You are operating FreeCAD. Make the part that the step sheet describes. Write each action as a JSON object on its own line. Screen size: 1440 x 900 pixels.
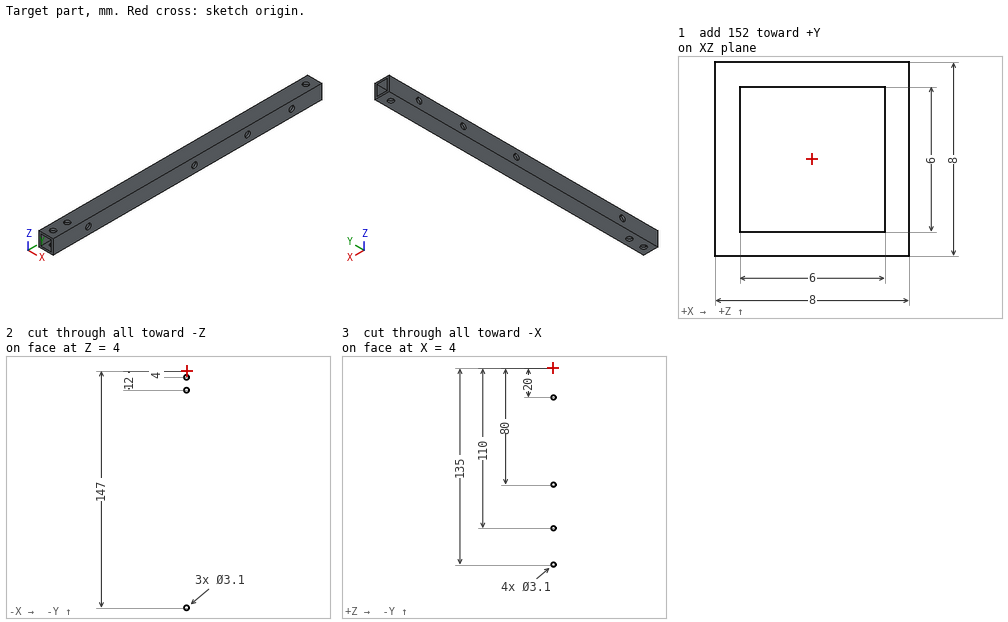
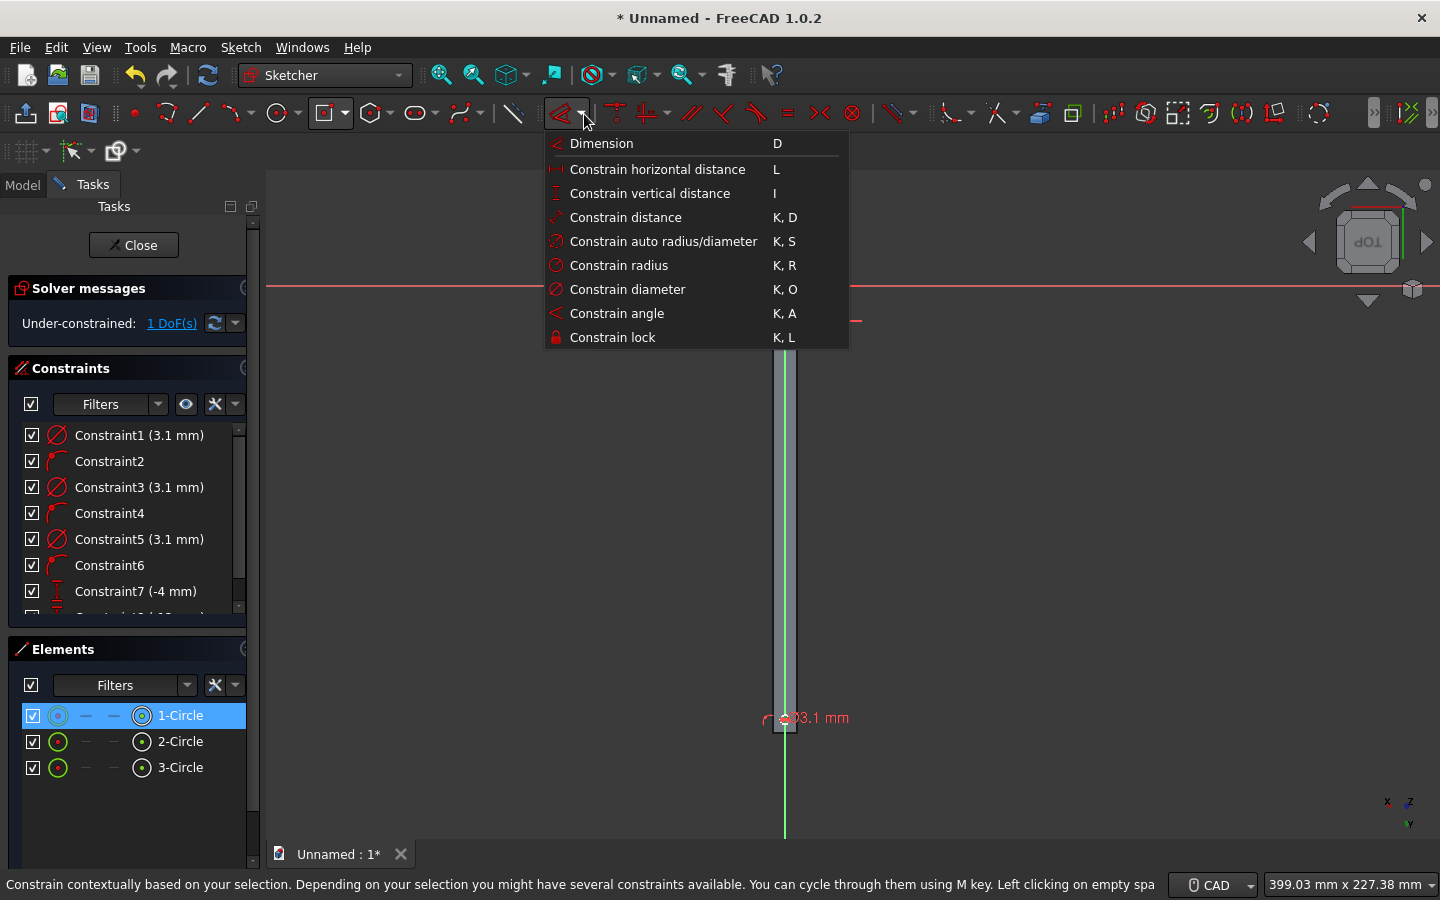
{"action": "left_click", "coordinate": [697, 193]}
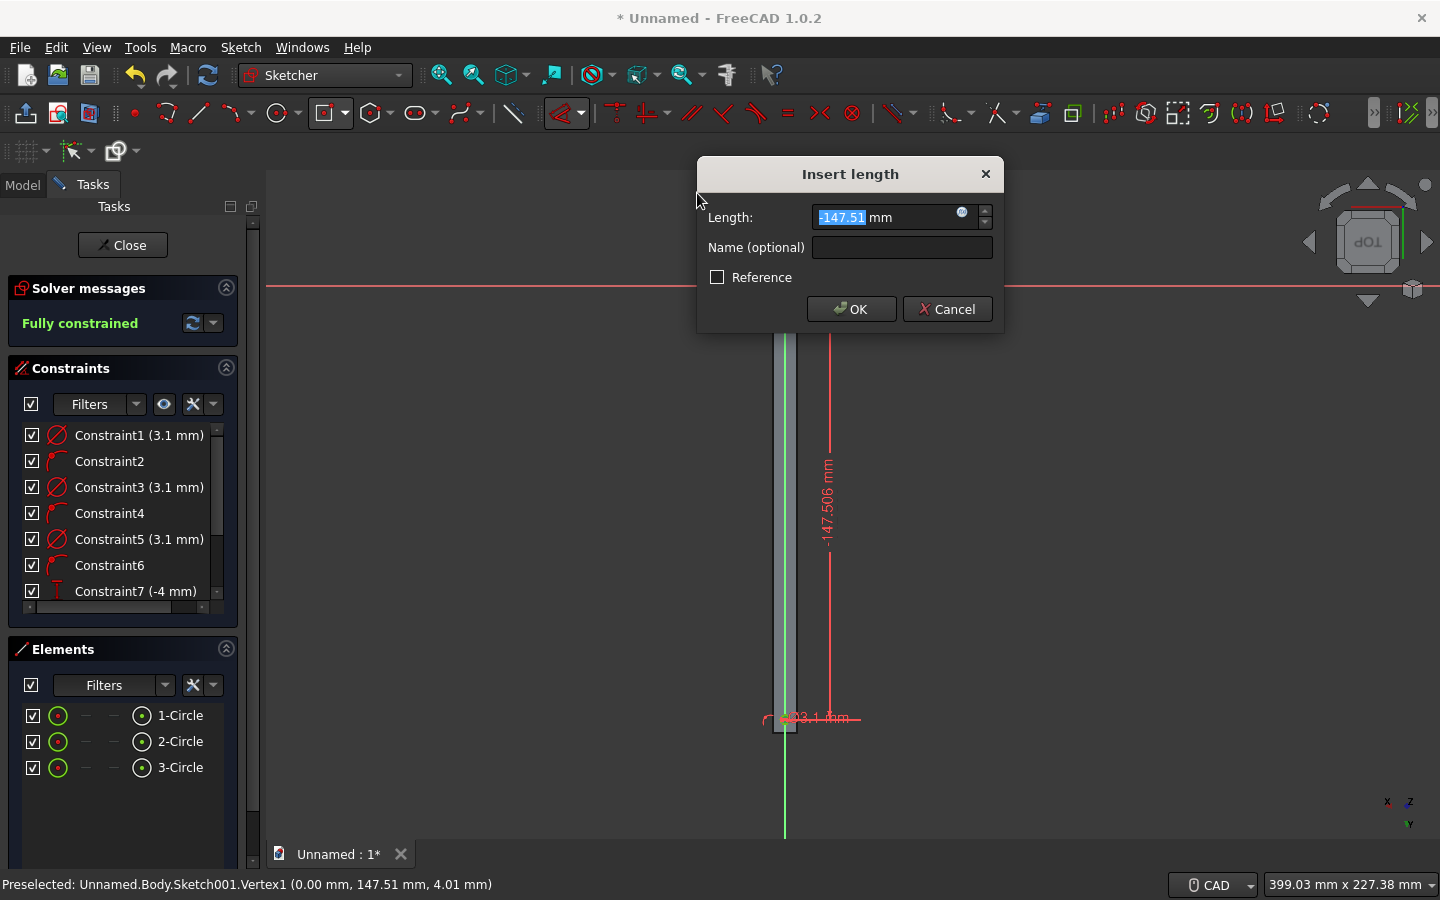
{"action": "type", "text": "-147"}
{"action": "key", "text": "Return"}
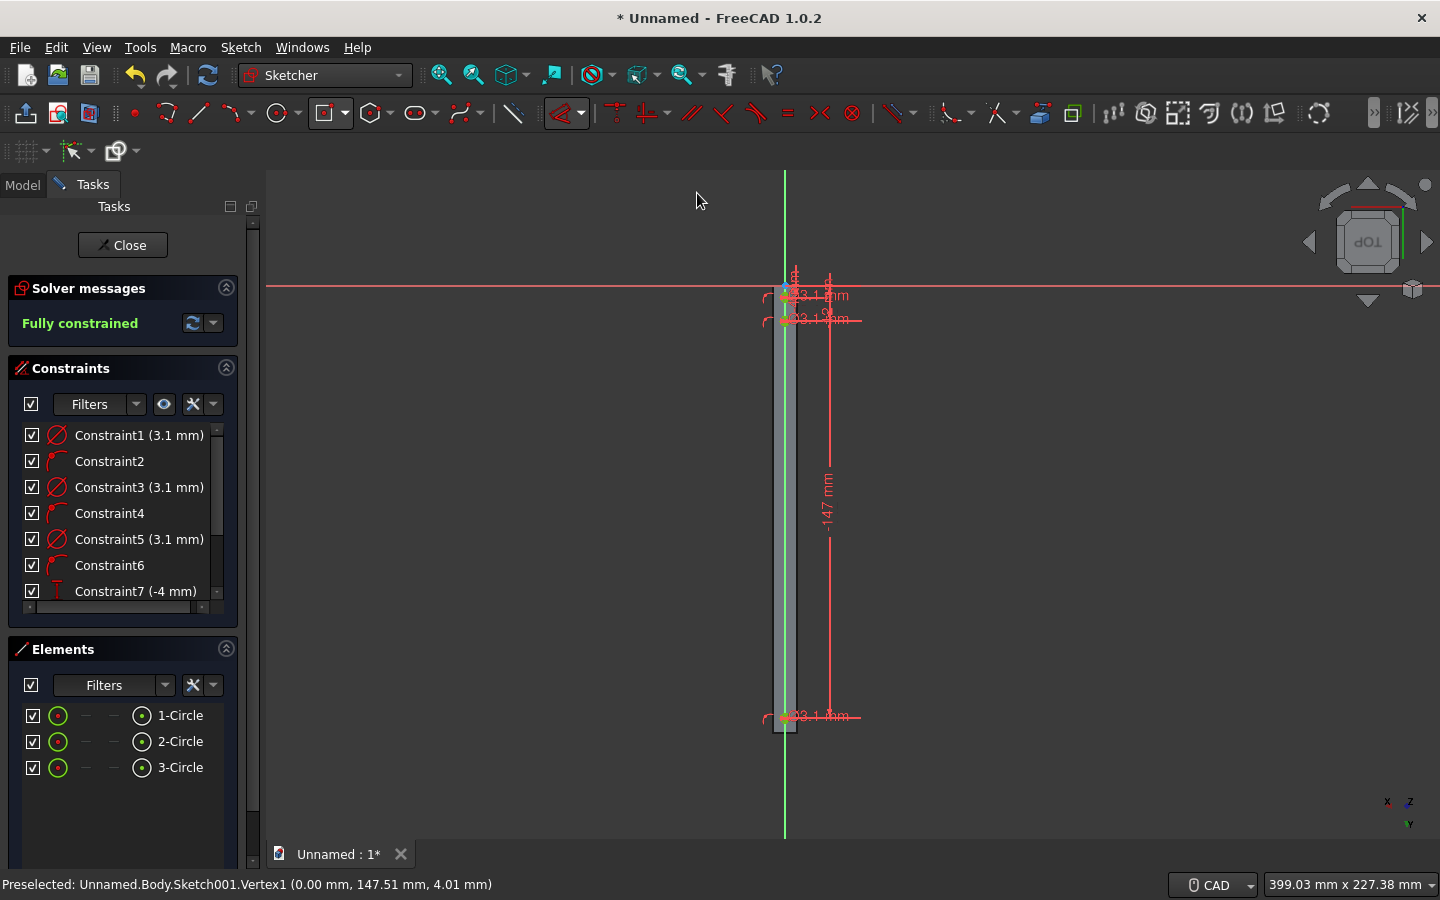
{"action": "left_click", "coordinate": [123, 245]}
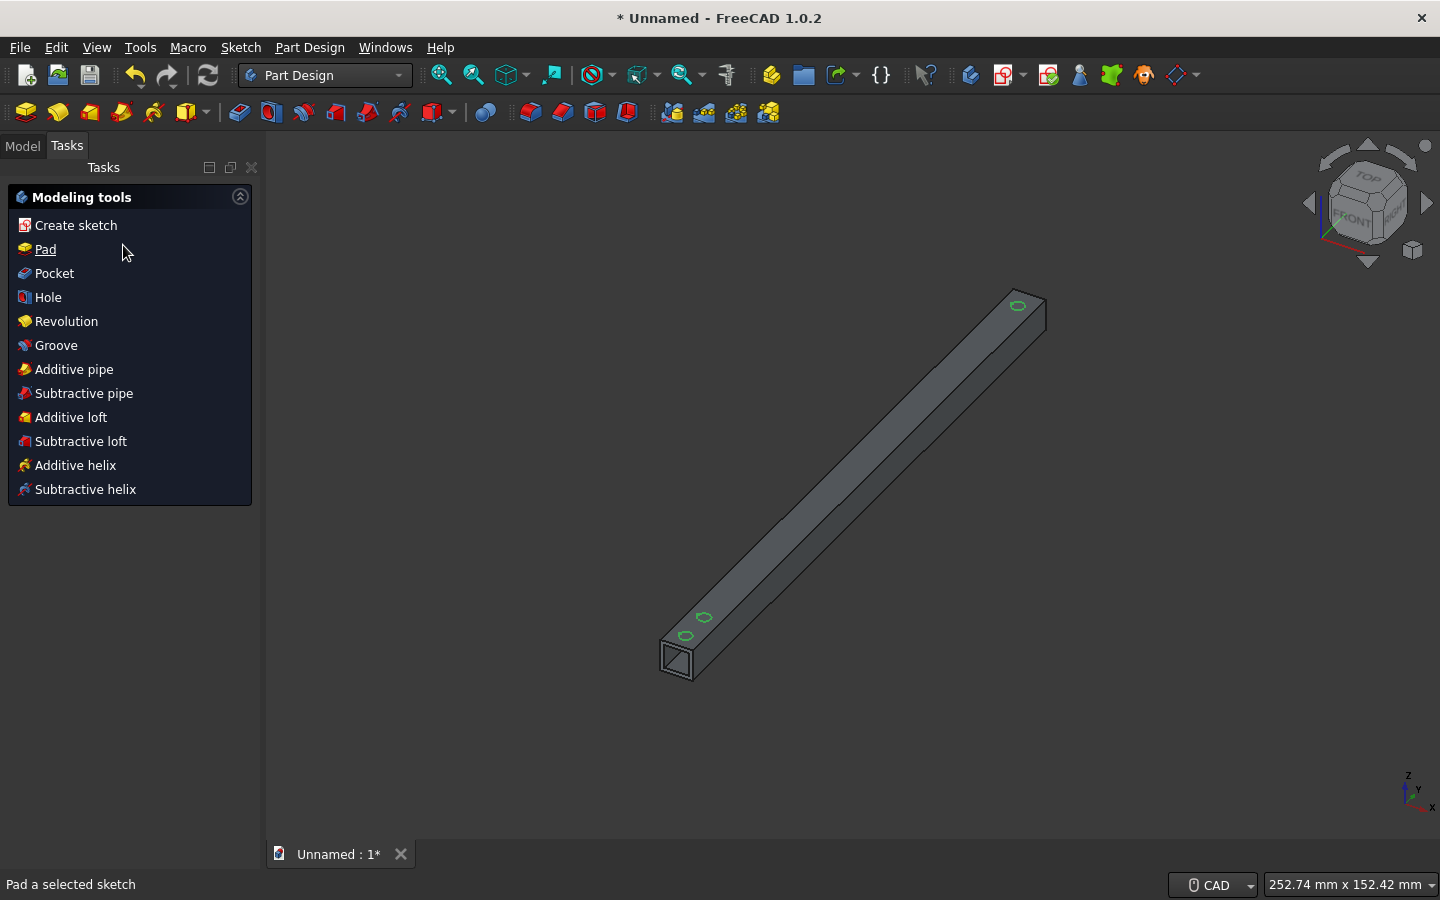
{"action": "left_click", "coordinate": [240, 112]}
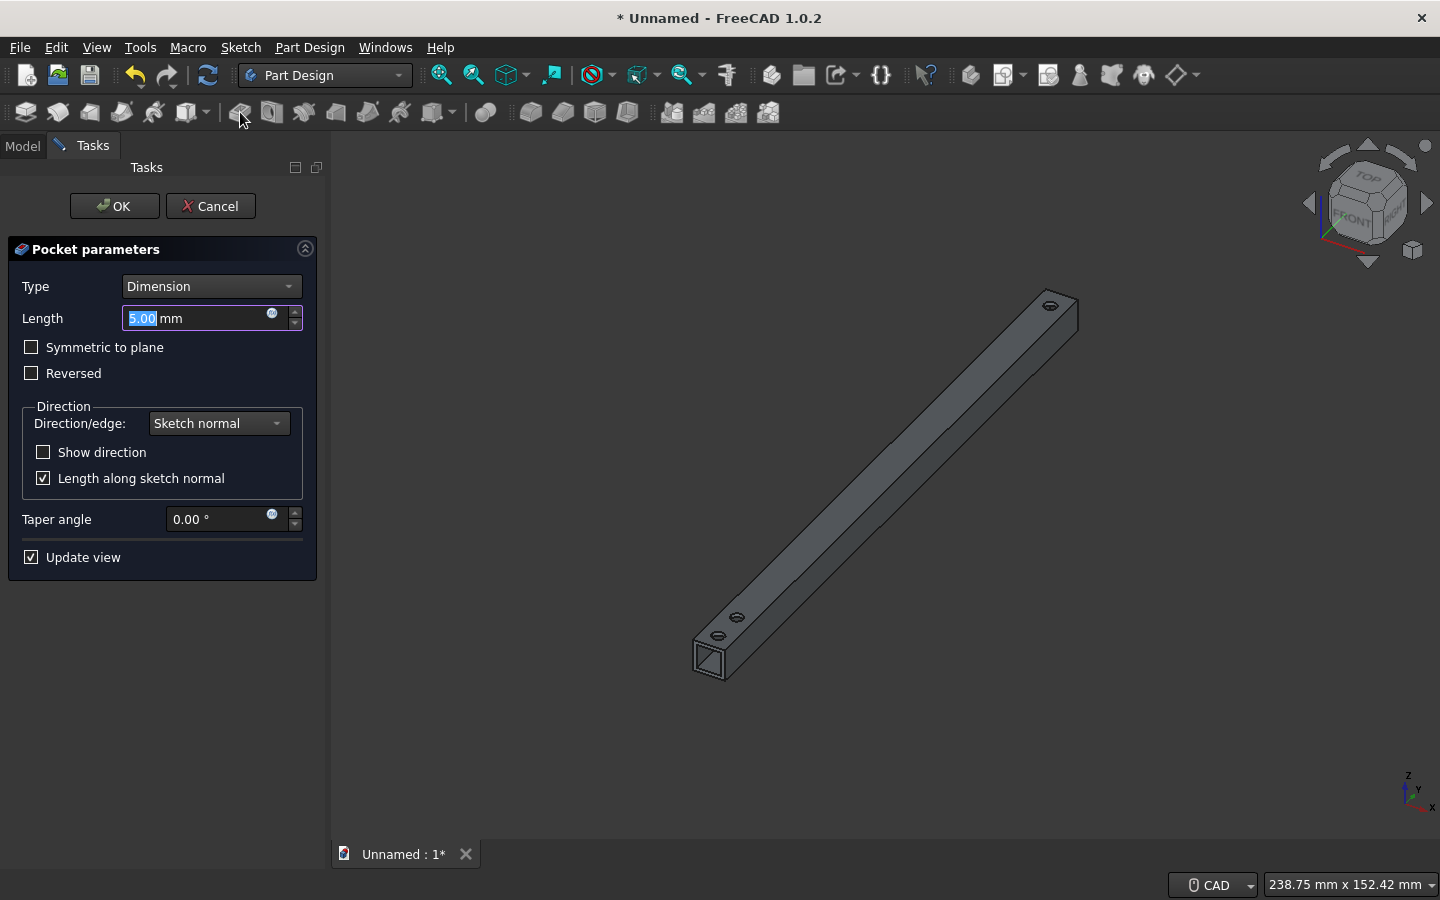
{"action": "left_click", "coordinate": [212, 286]}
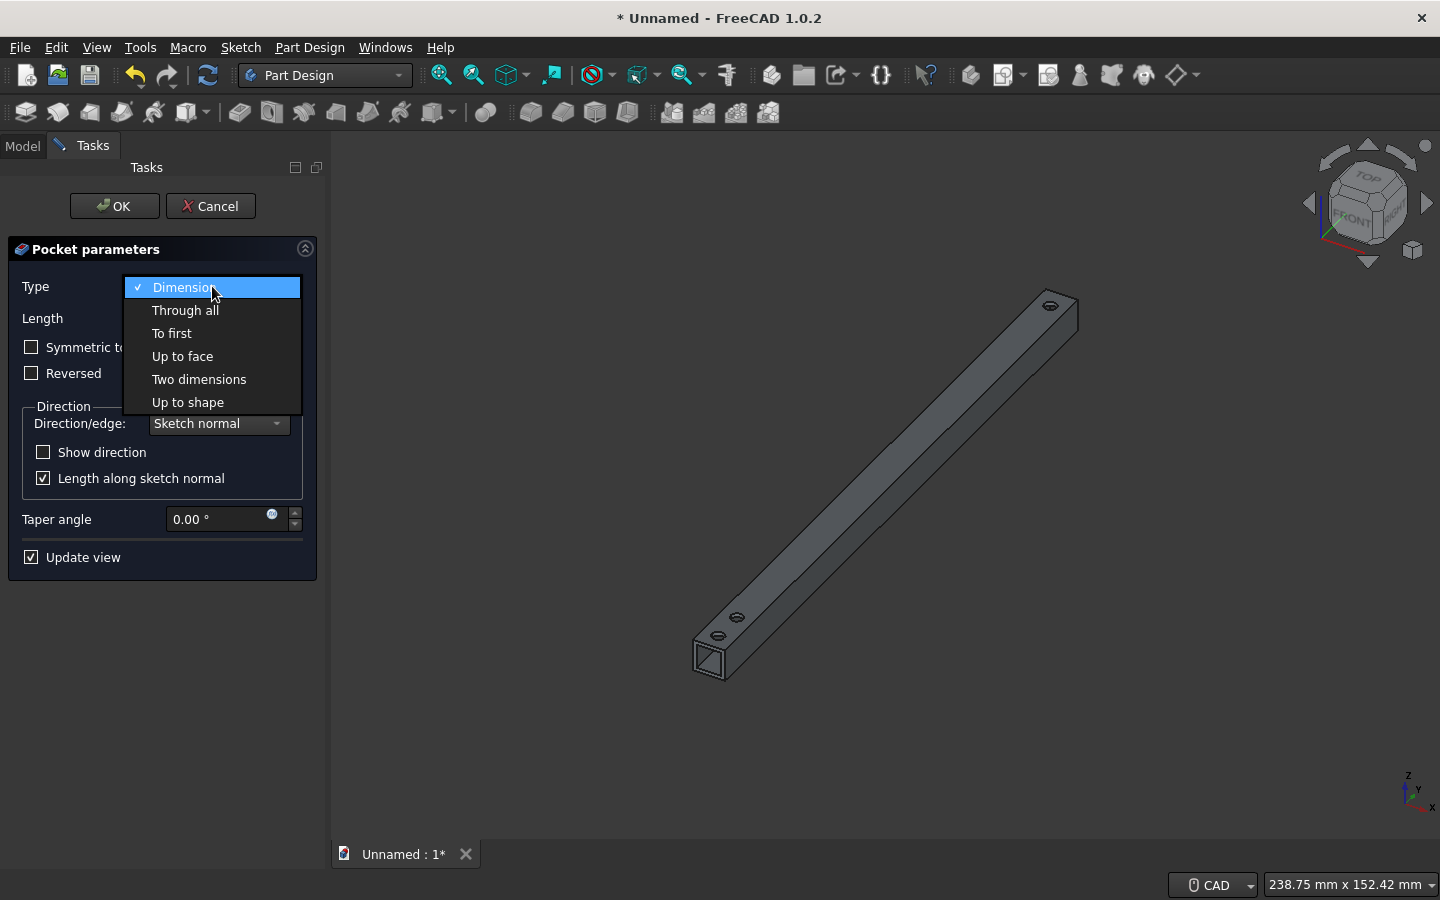
{"action": "left_click", "coordinate": [212, 310]}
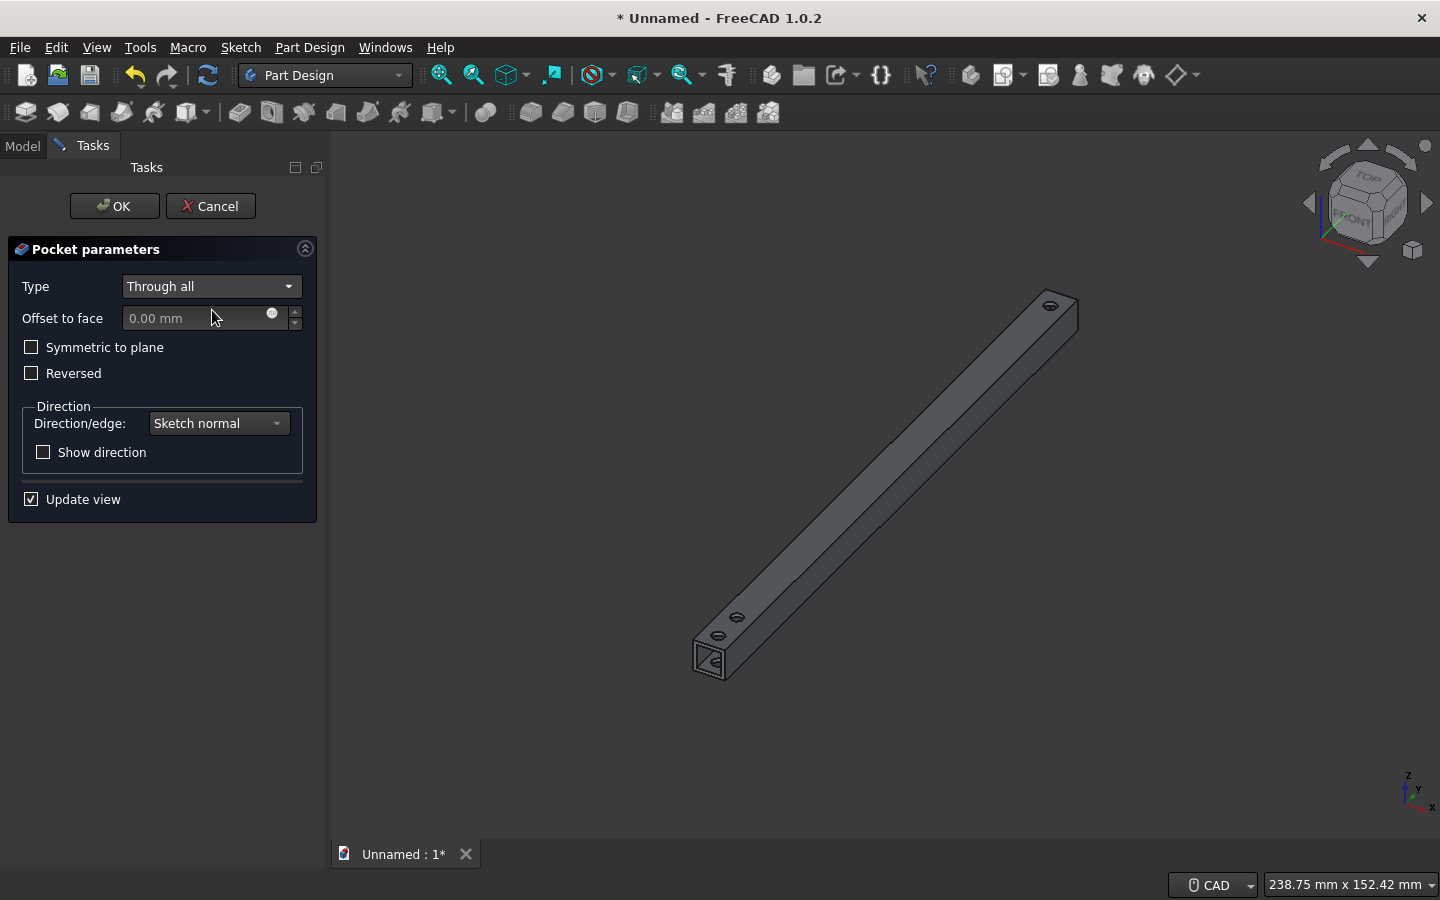
{"action": "left_click", "coordinate": [115, 206]}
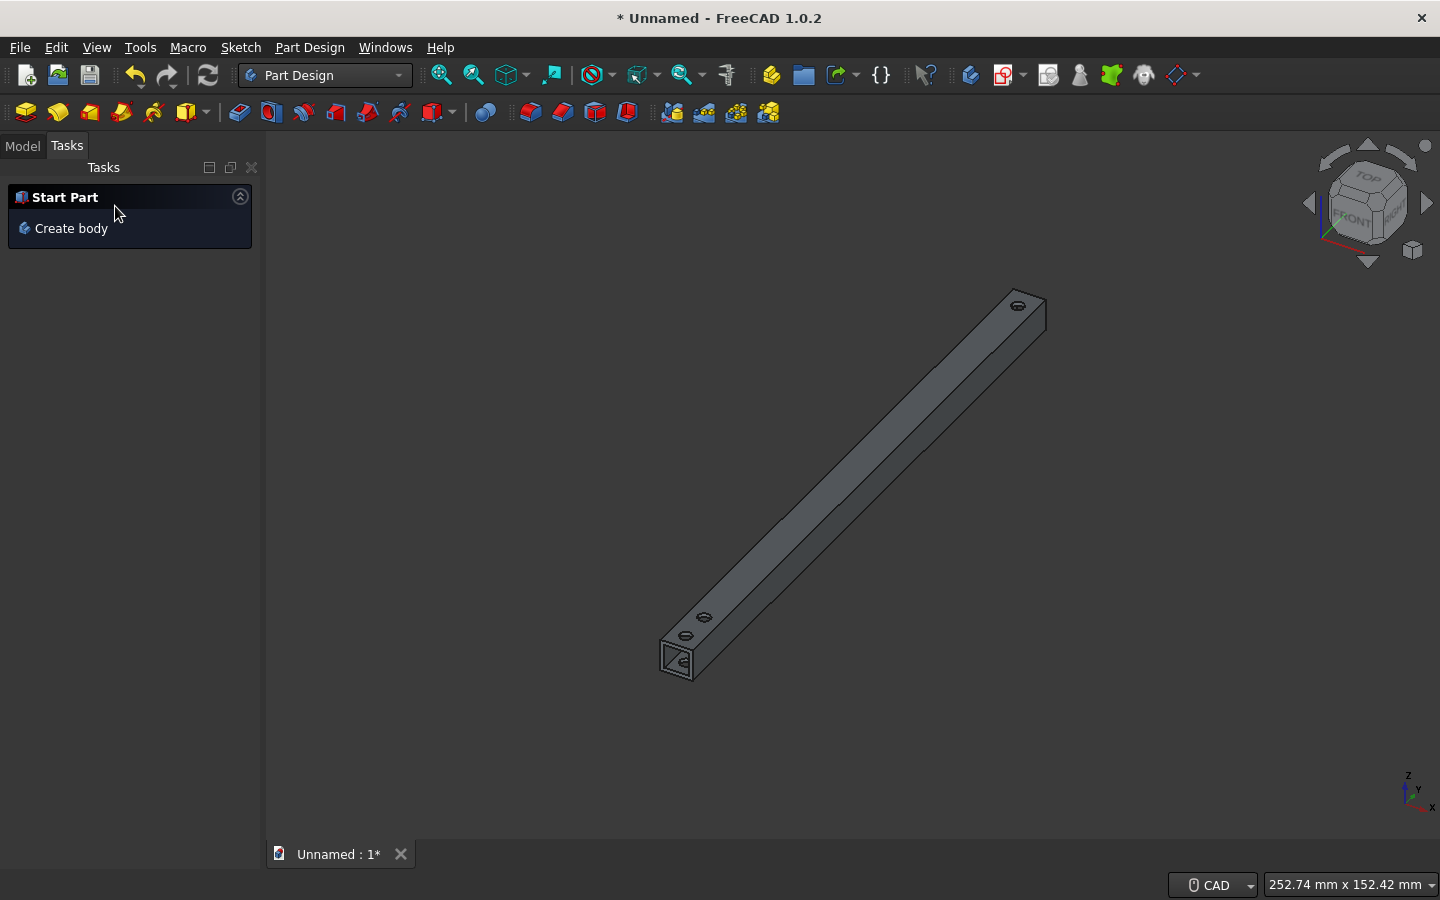
{"action": "left_click", "coordinate": [1020, 339]}